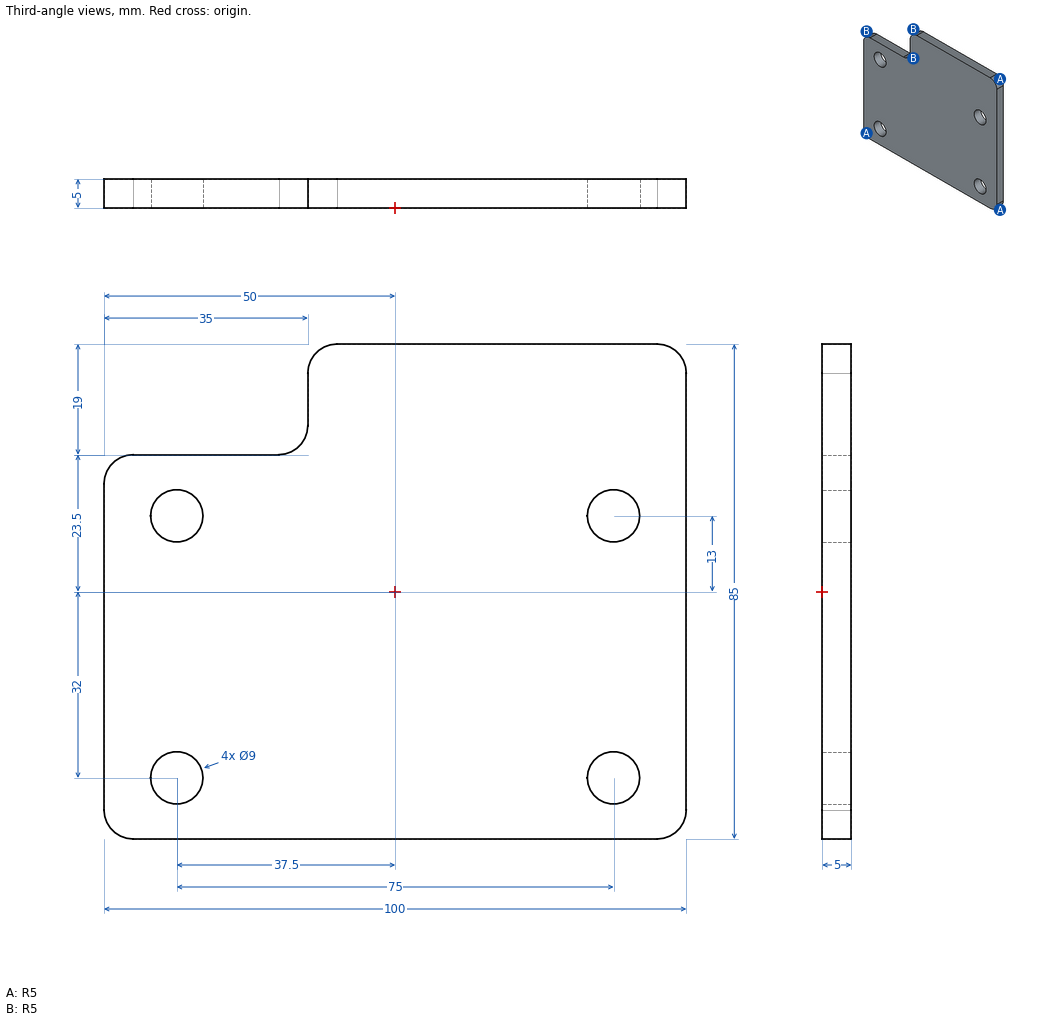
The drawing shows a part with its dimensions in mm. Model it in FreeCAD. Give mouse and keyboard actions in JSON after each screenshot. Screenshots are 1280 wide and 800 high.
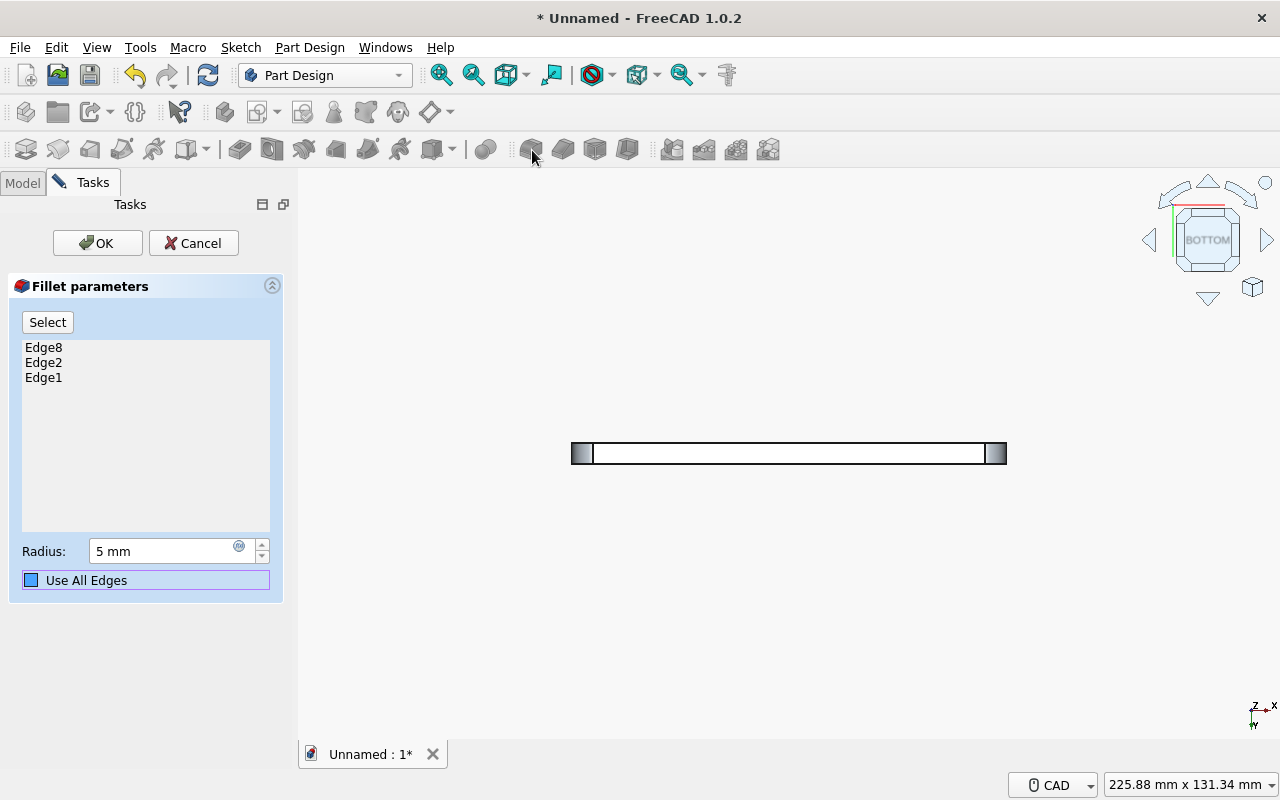
{"action": "left_click", "coordinate": [98, 243]}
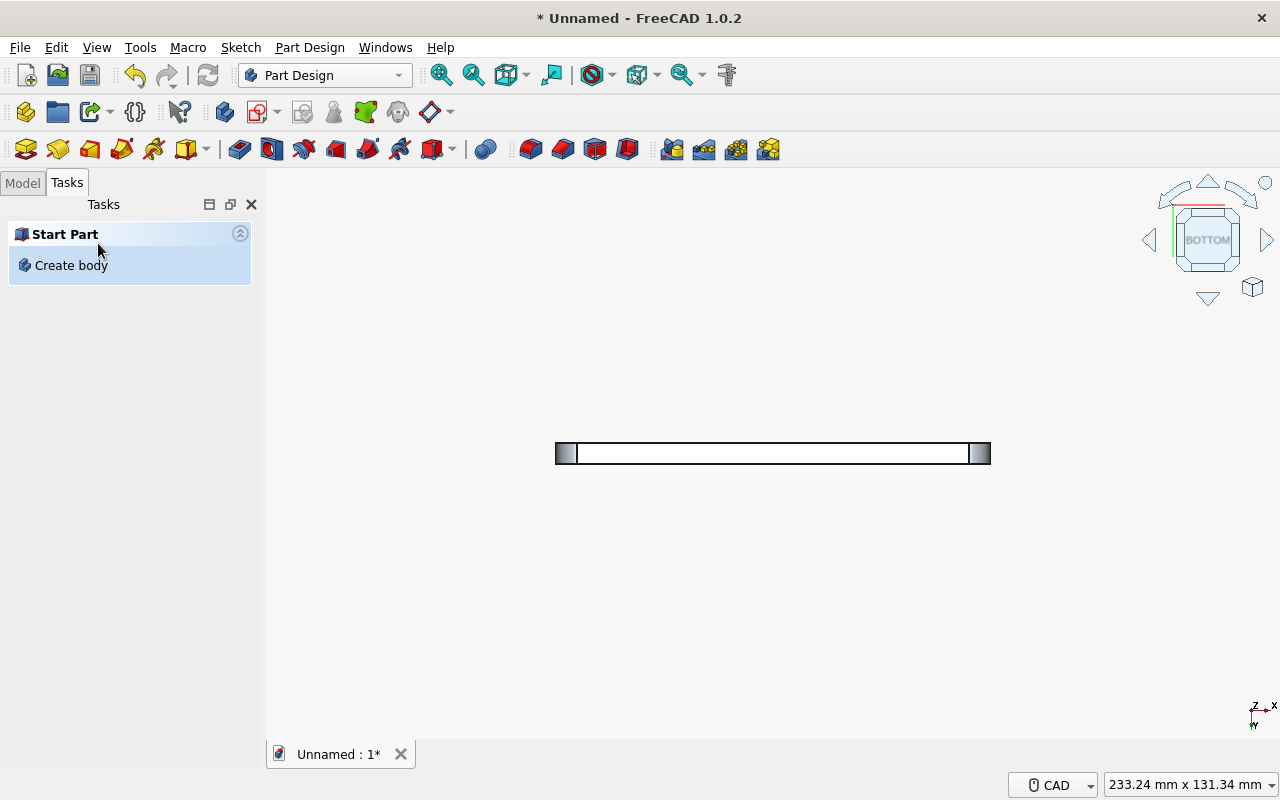
{"action": "left_click", "coordinate": [442, 76]}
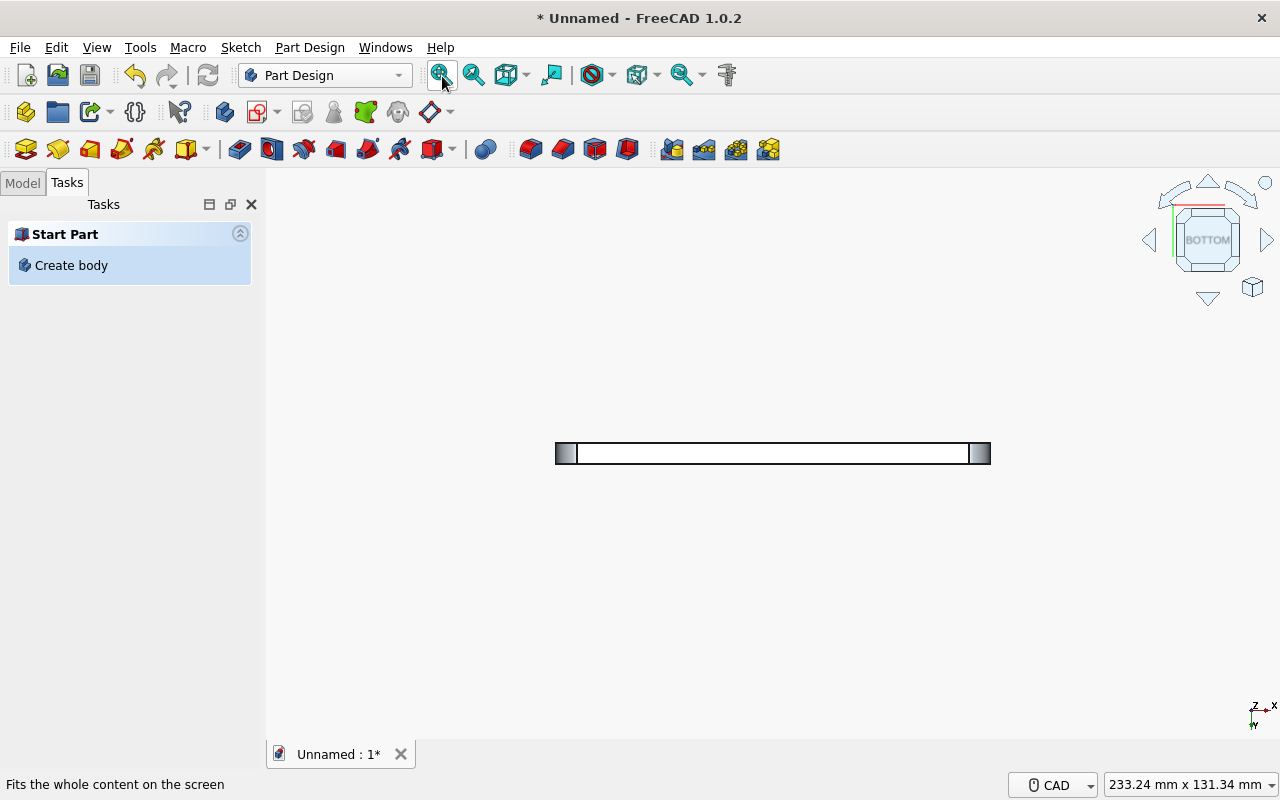
{"action": "key", "text": "4"}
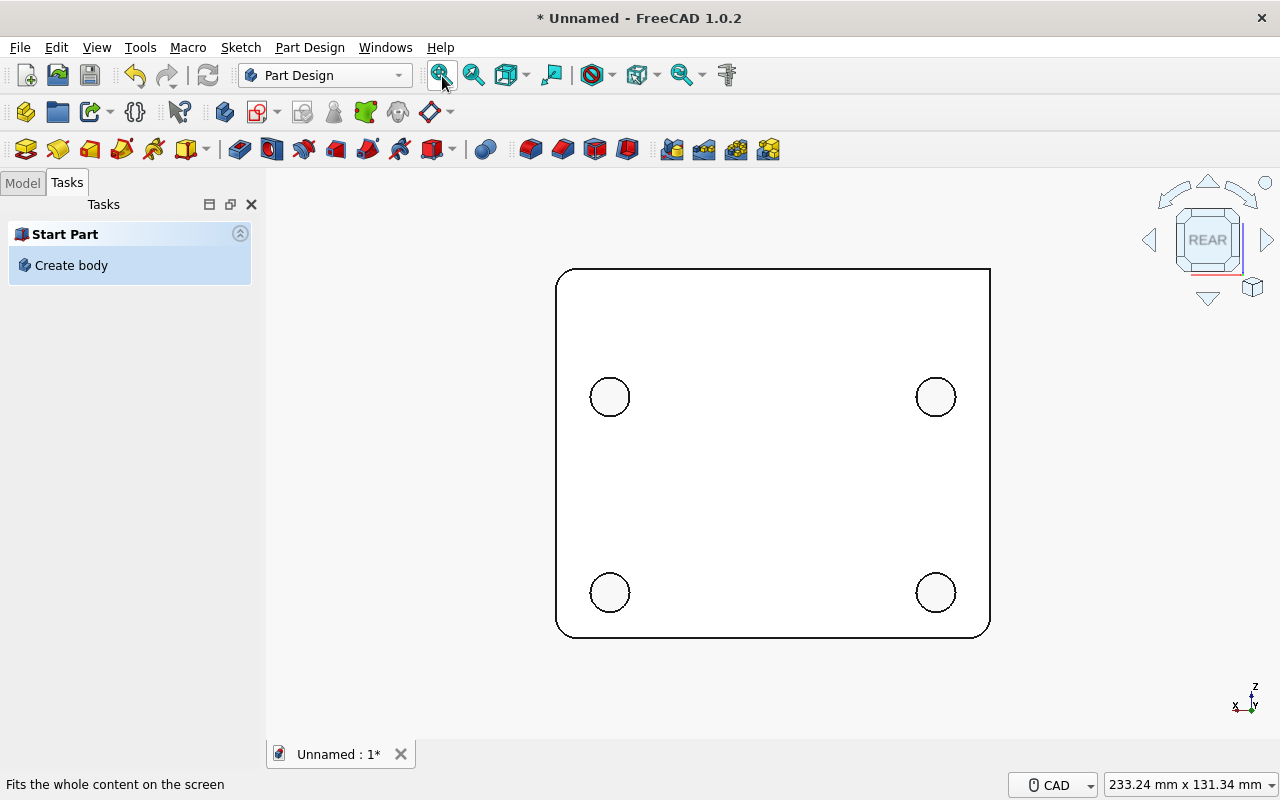
{"action": "left_click", "coordinate": [773, 453]}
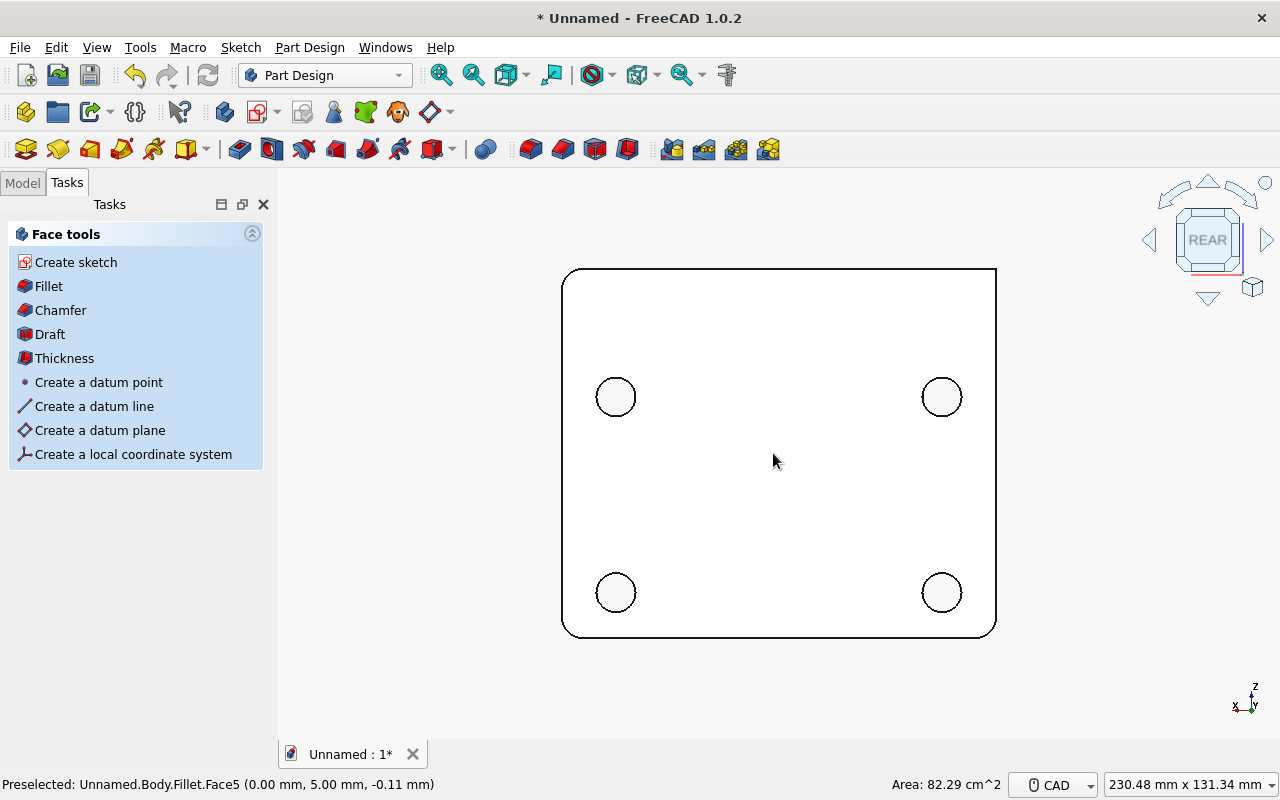
{"action": "left_click", "coordinate": [258, 112]}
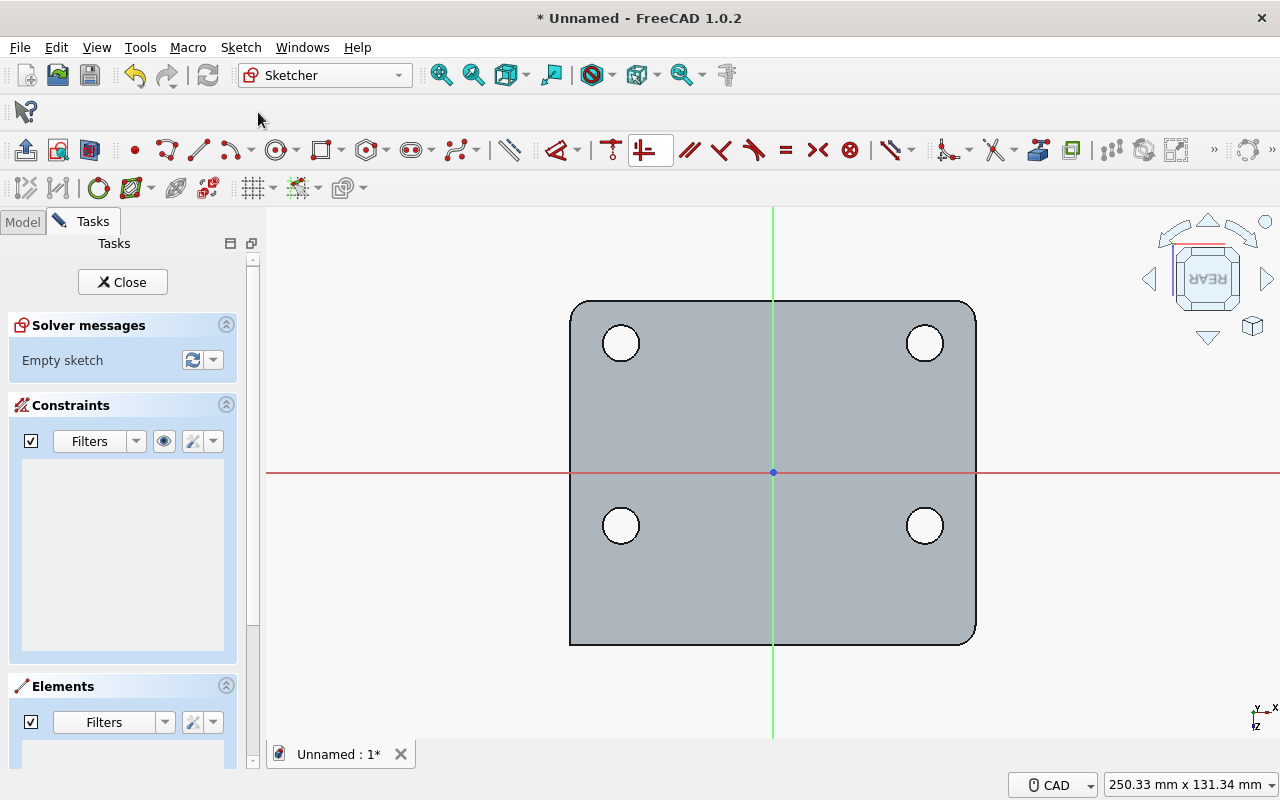
{"action": "scroll", "coordinate": [632, 664], "scroll_direction": "up", "scroll_amount": 3}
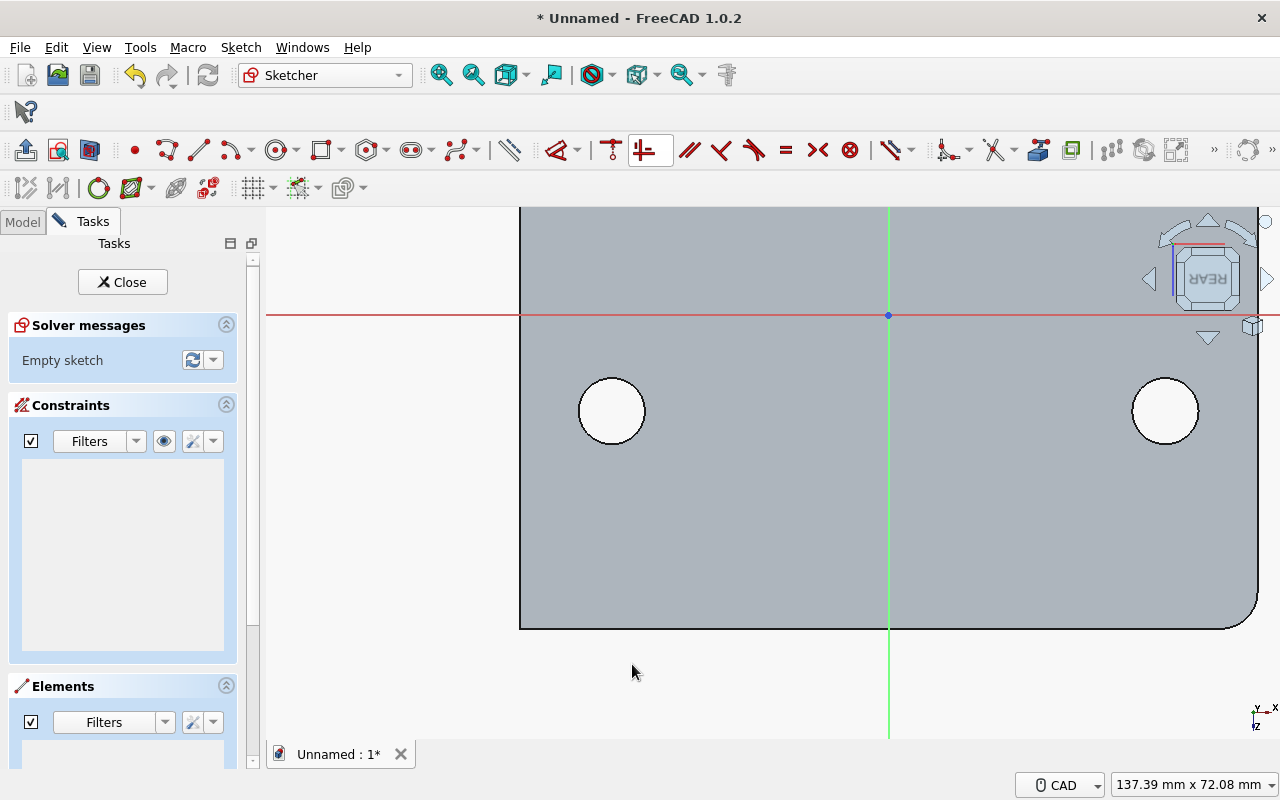
{"action": "left_click", "coordinate": [322, 150]}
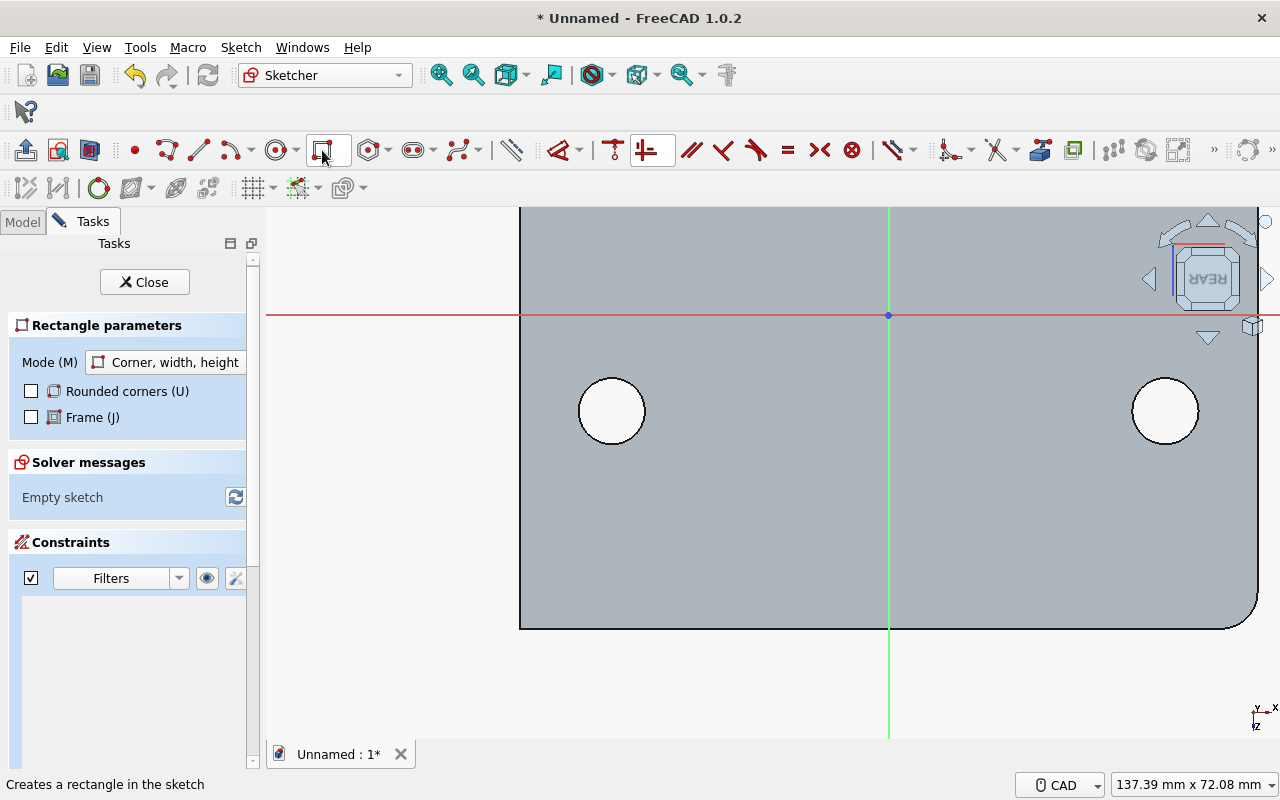
{"action": "left_click", "coordinate": [520, 489]}
{"action": "mouse_move", "coordinate": [778, 629]}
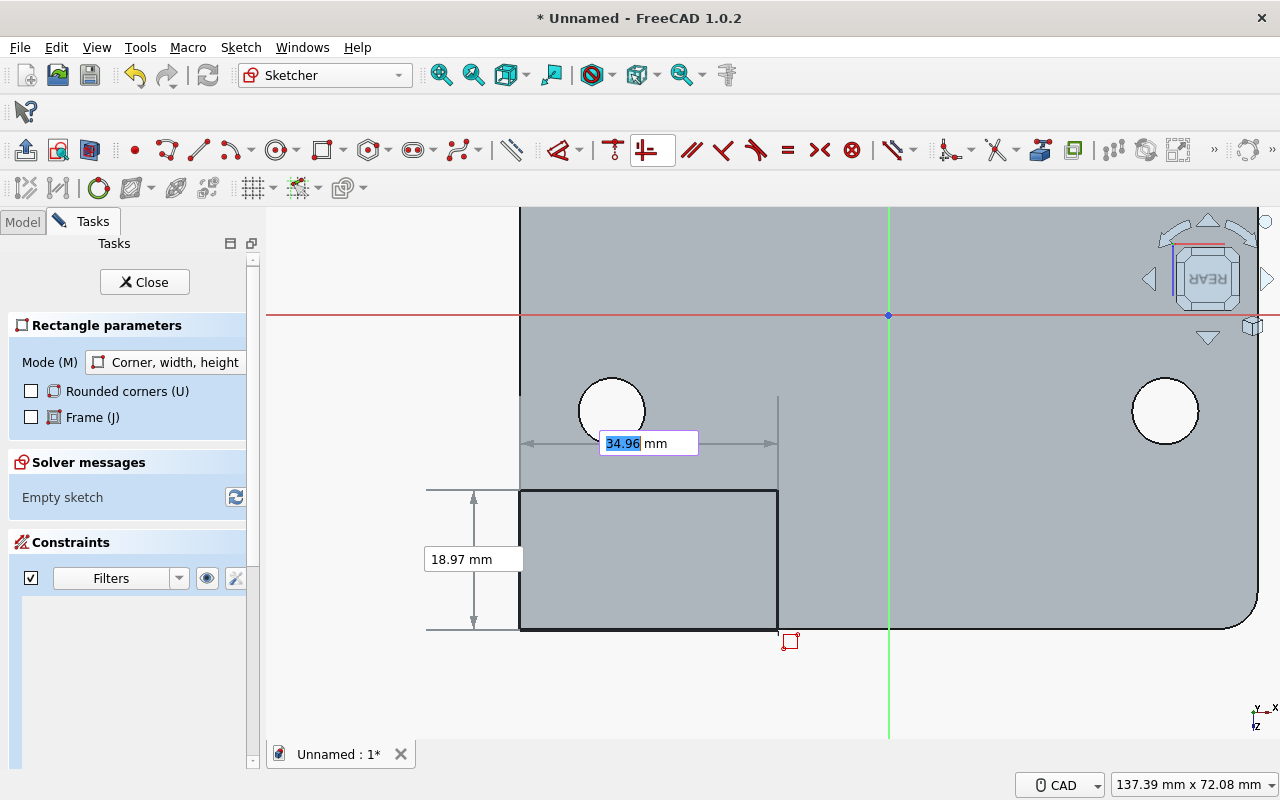
{"action": "type", "text": "35"}
{"action": "key", "text": "Tab"}
{"action": "type", "text": "19"}
{"action": "key", "text": "Return"}
{"action": "key", "text": "Escape"}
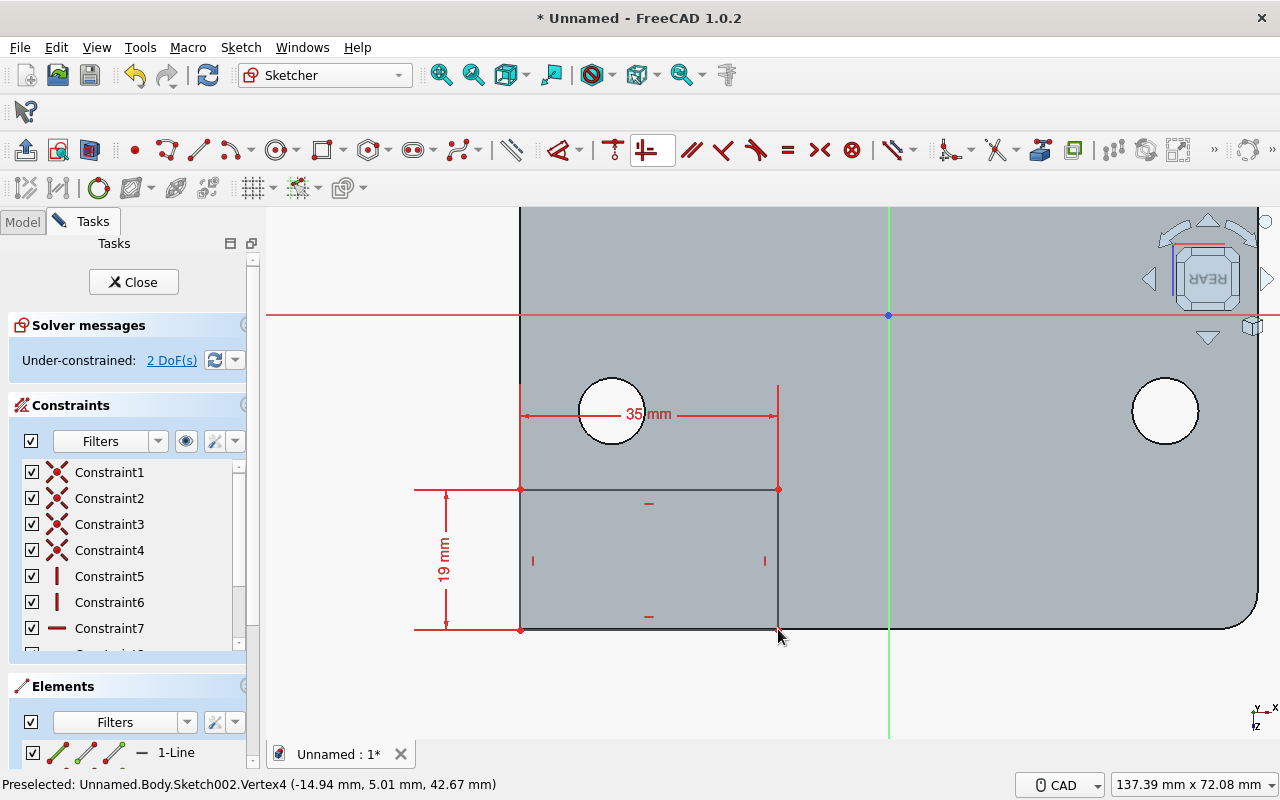
{"action": "left_click", "coordinate": [558, 150]}